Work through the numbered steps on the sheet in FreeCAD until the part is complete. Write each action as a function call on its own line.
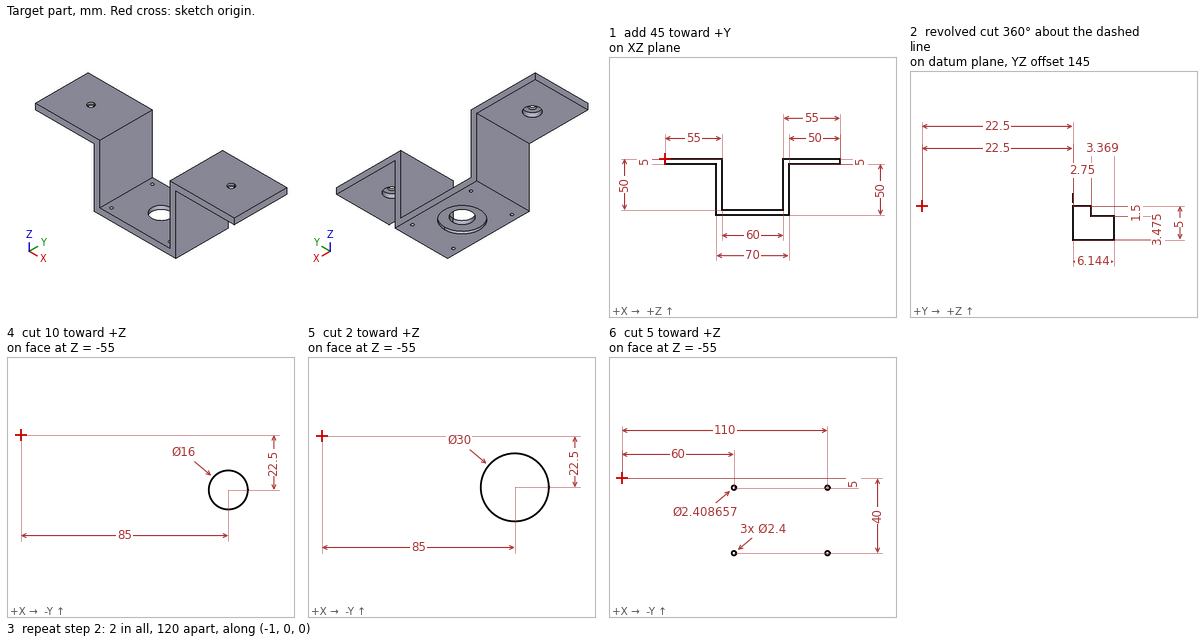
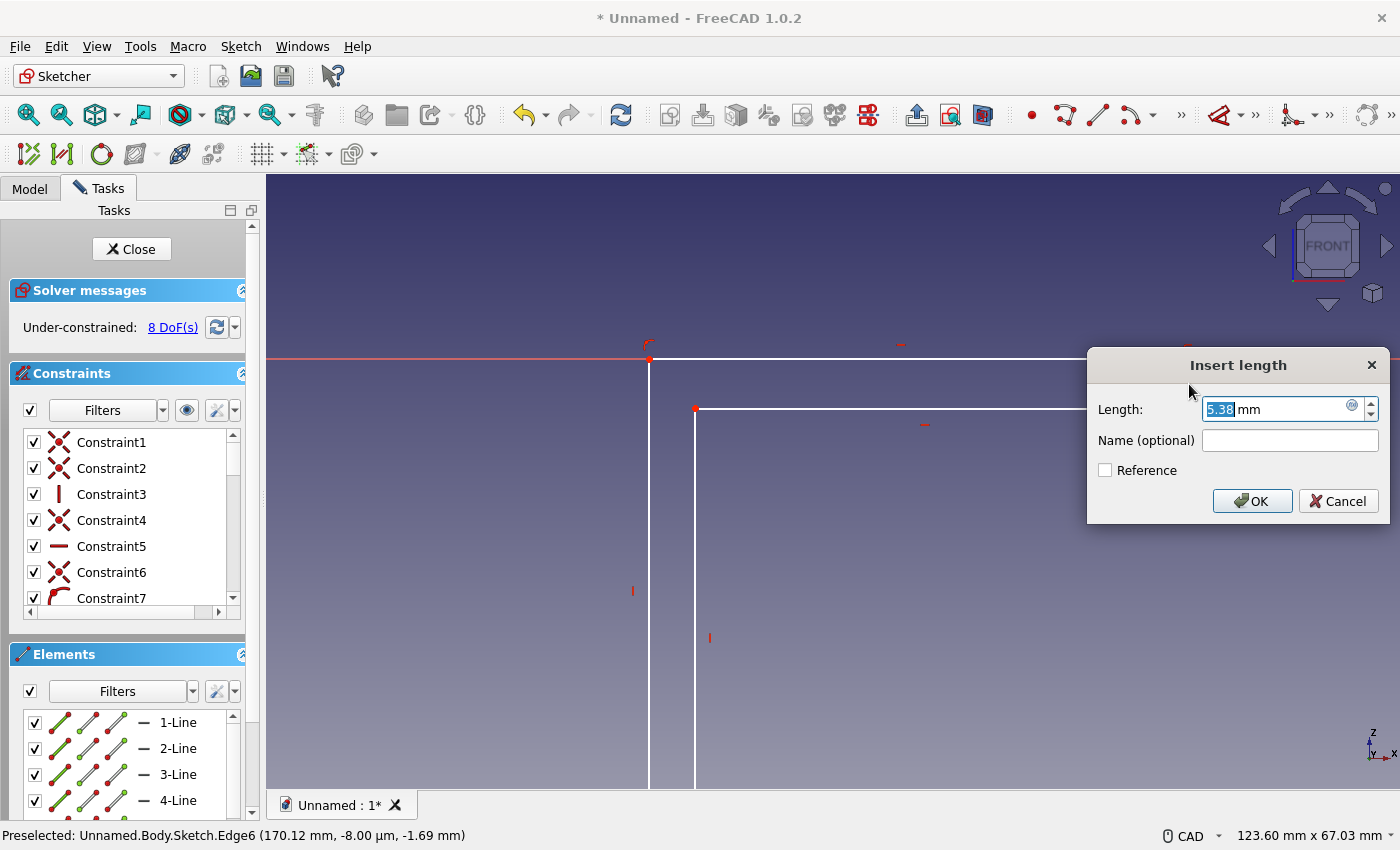
text(5)
key(Return)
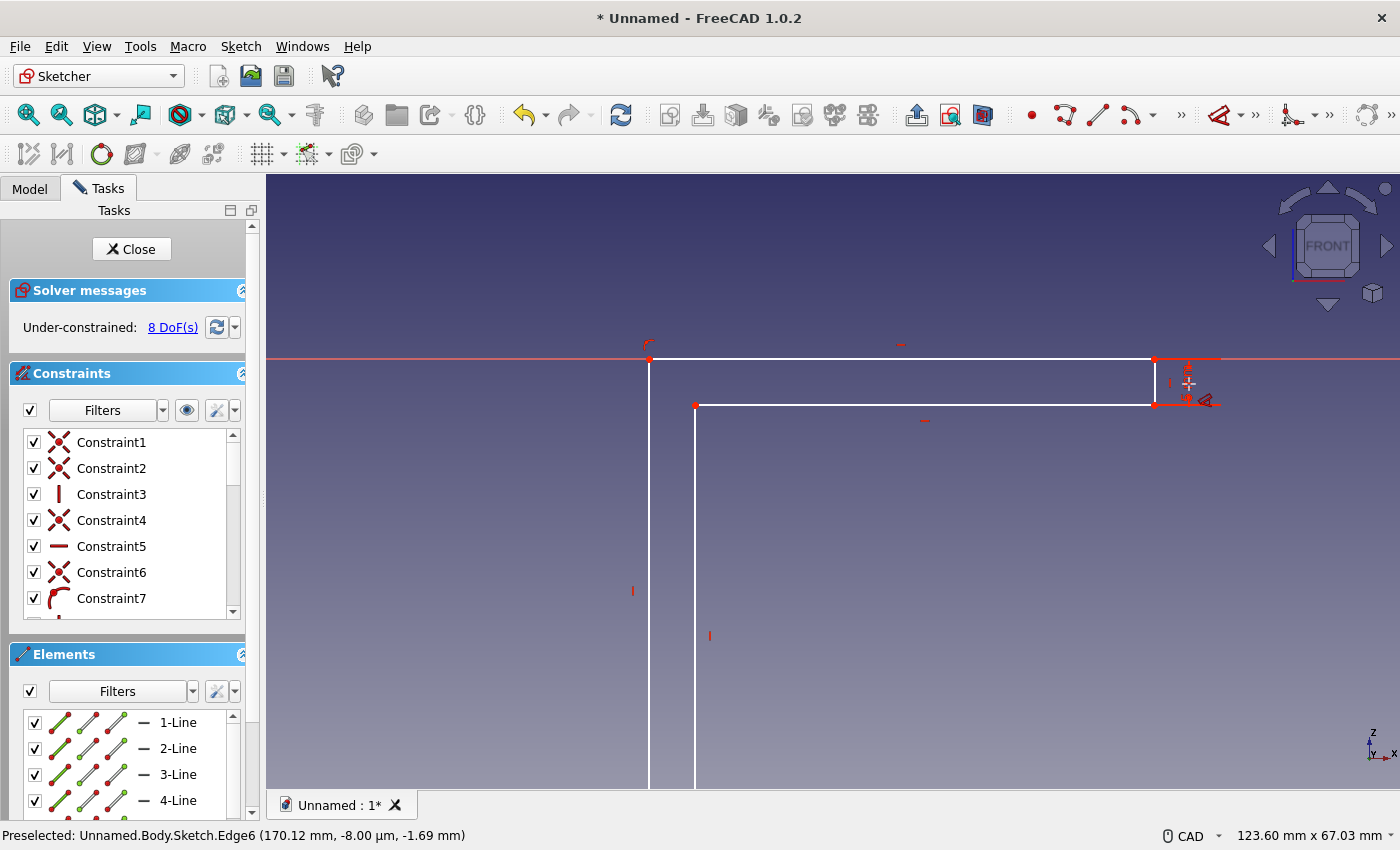
scroll(1083, 375, down, 4)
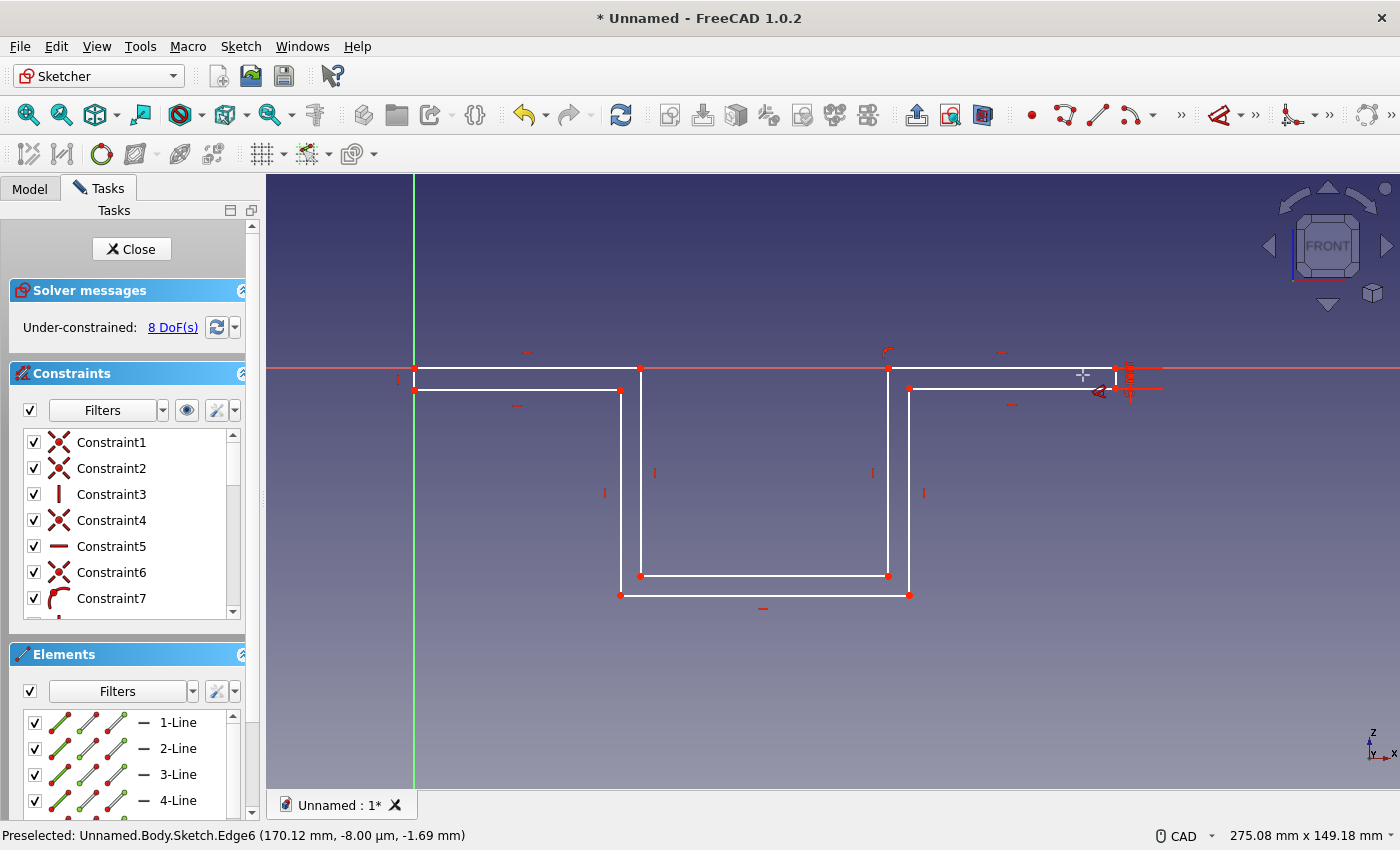
scroll(414, 384, up, 4)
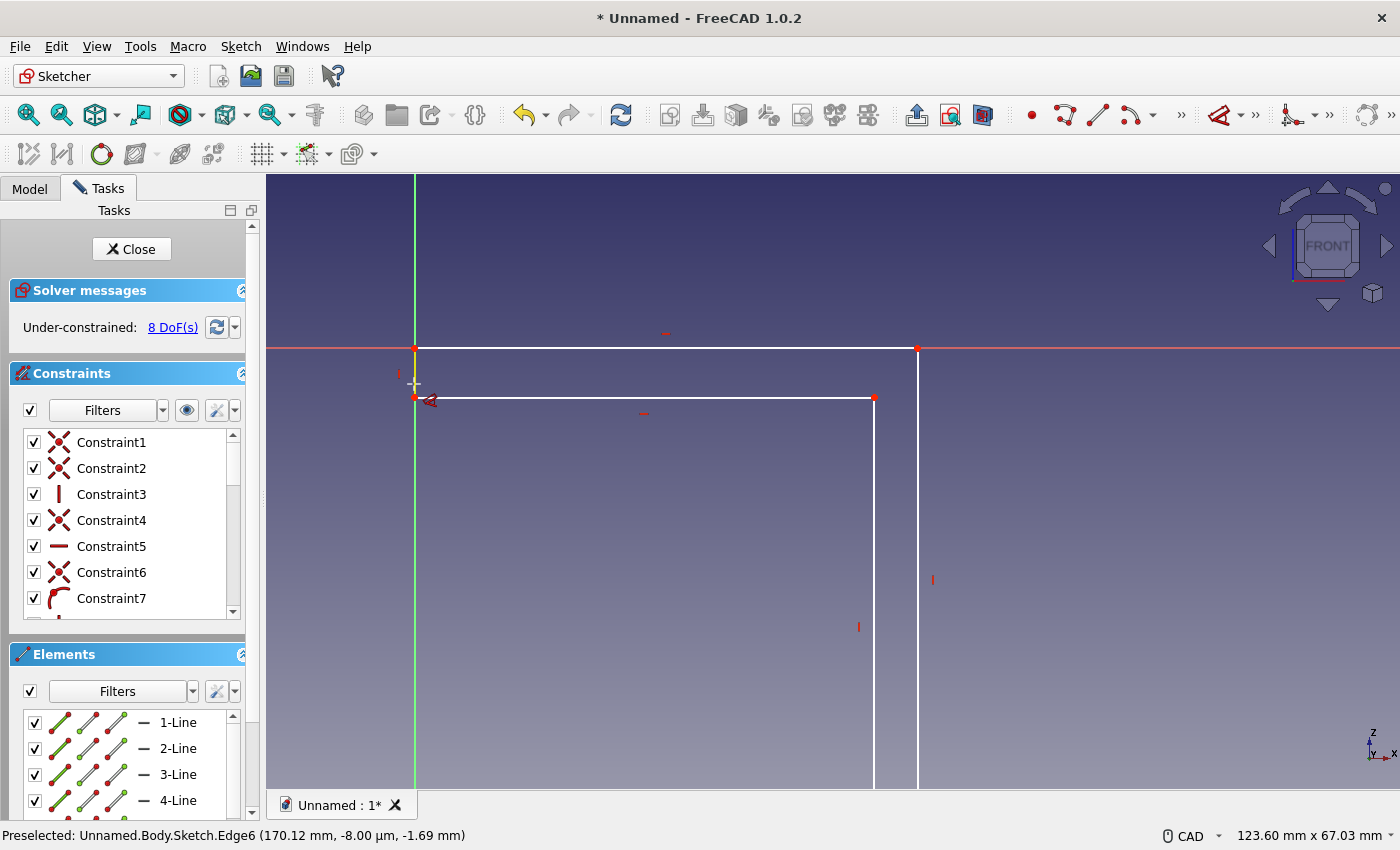
click(415, 383)
click(381, 373)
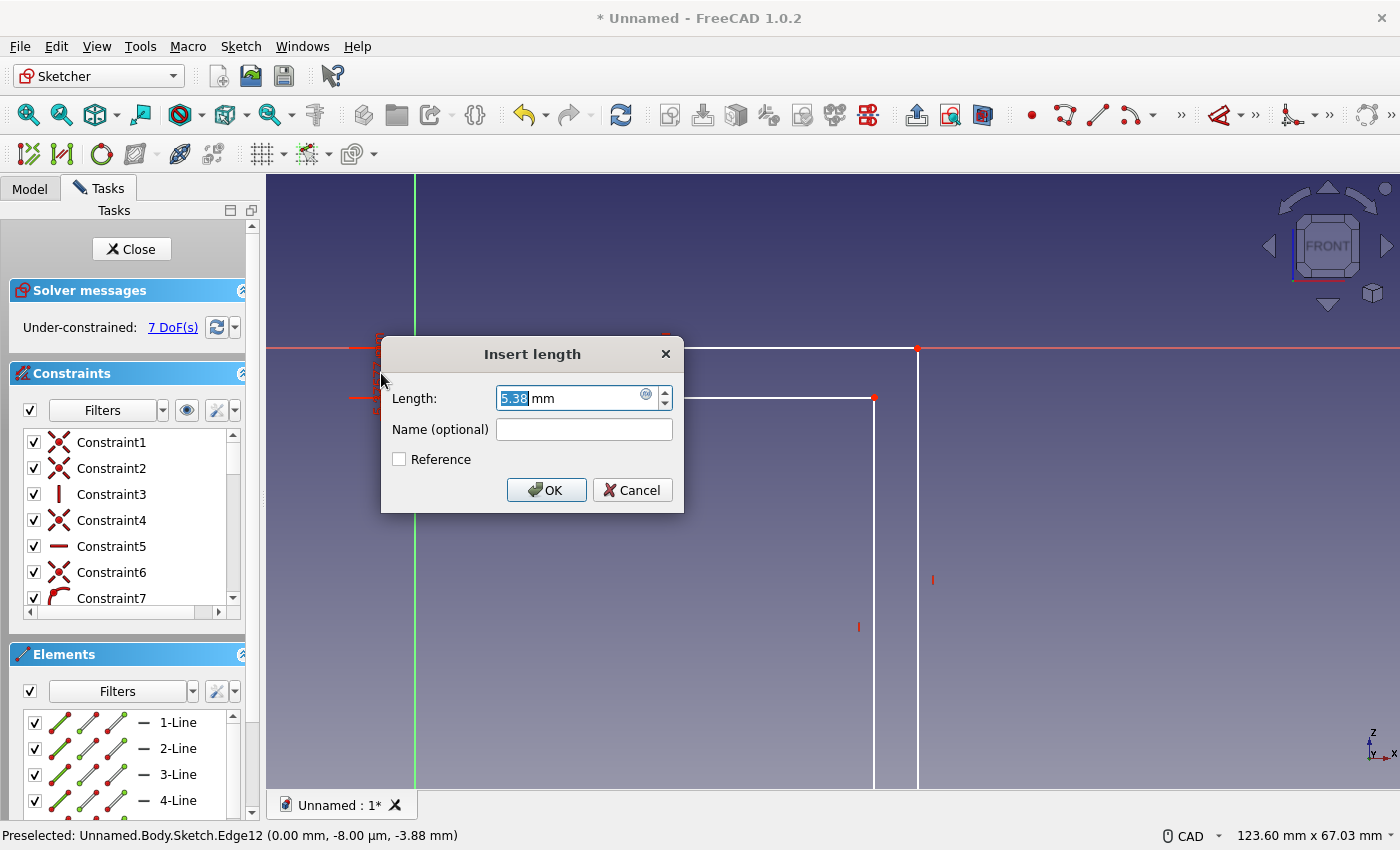
text(5)
key(Return)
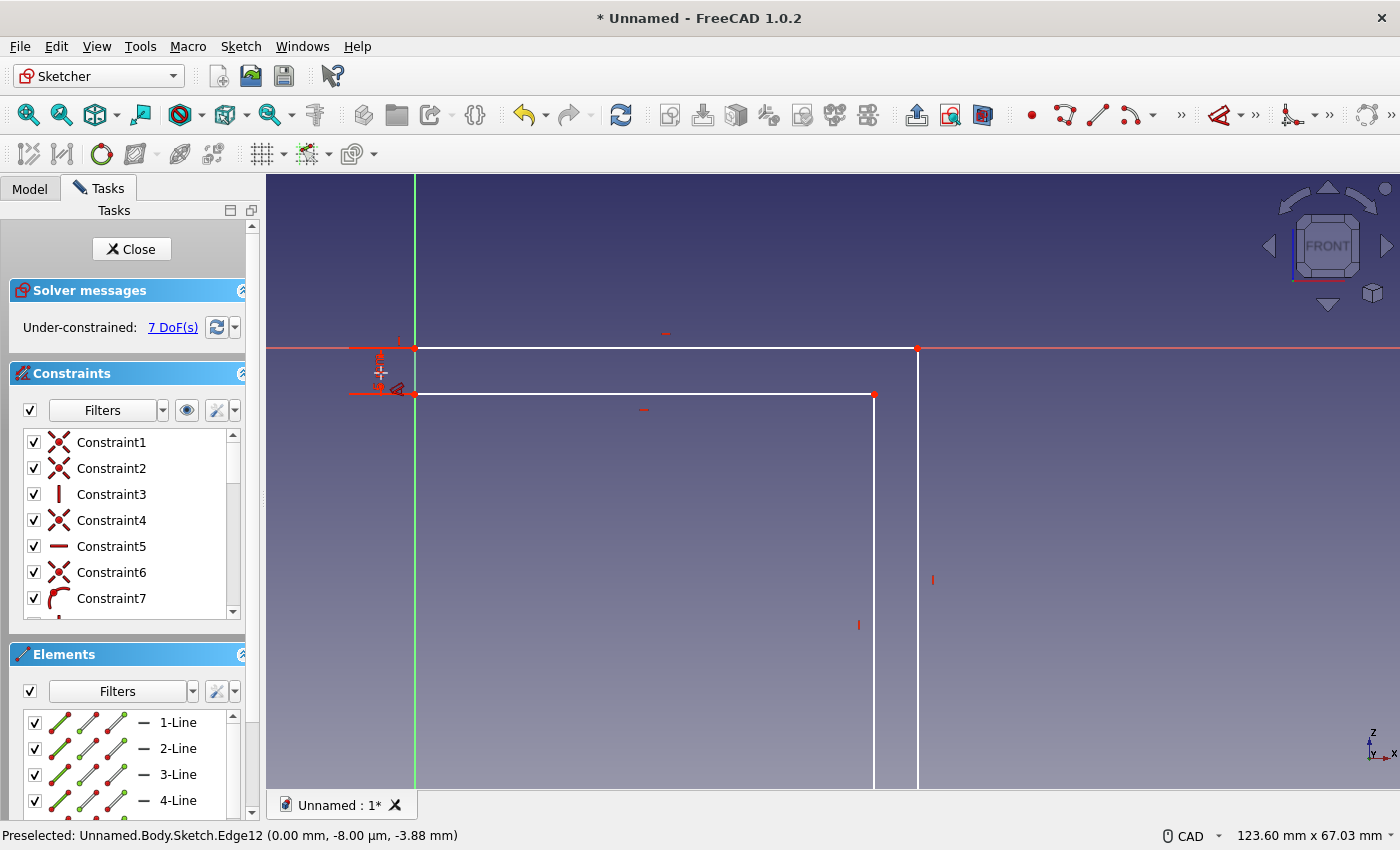
click(566, 348)
click(666, 314)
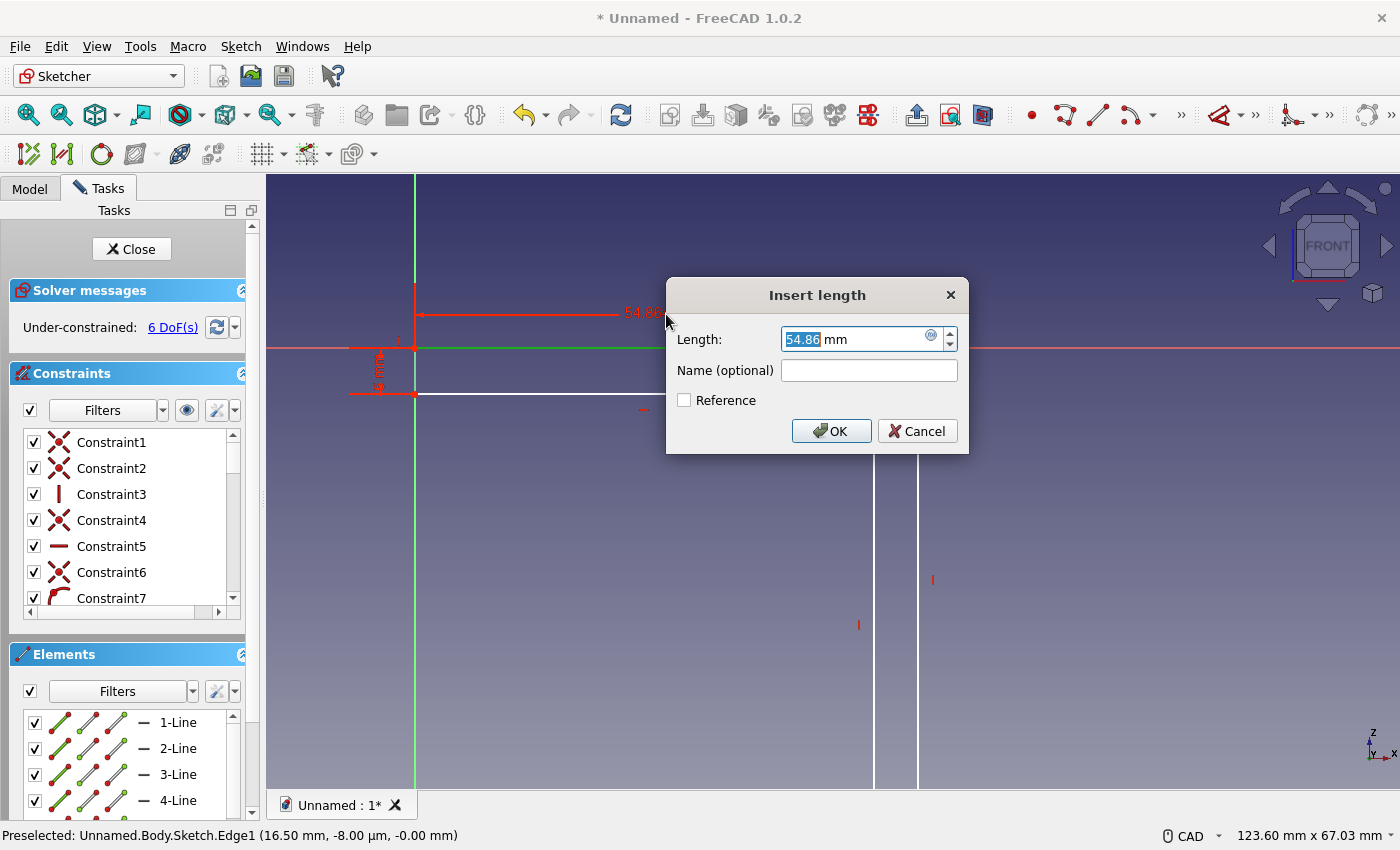
text(55)
key(Return)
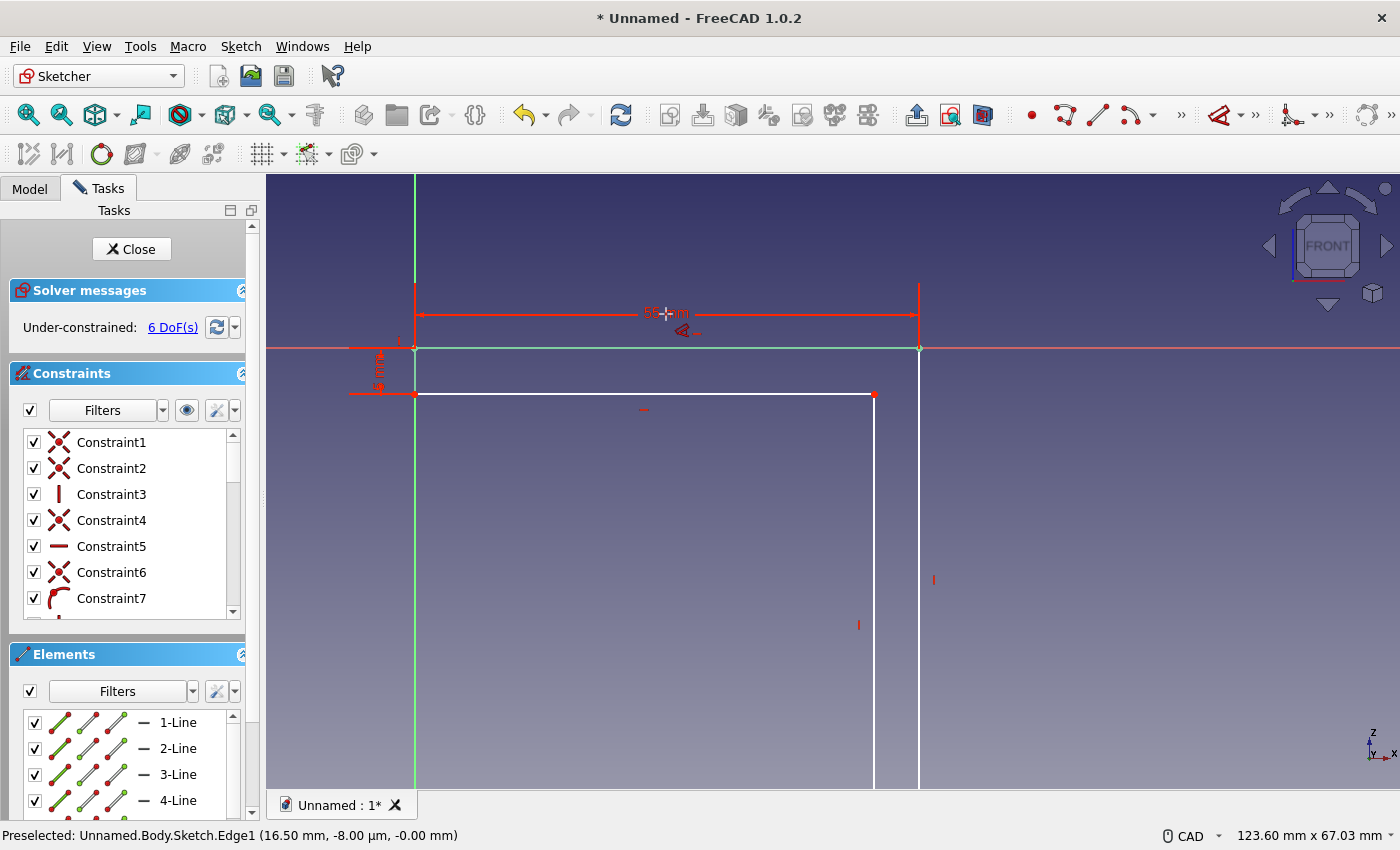
click(919, 487)
click(953, 555)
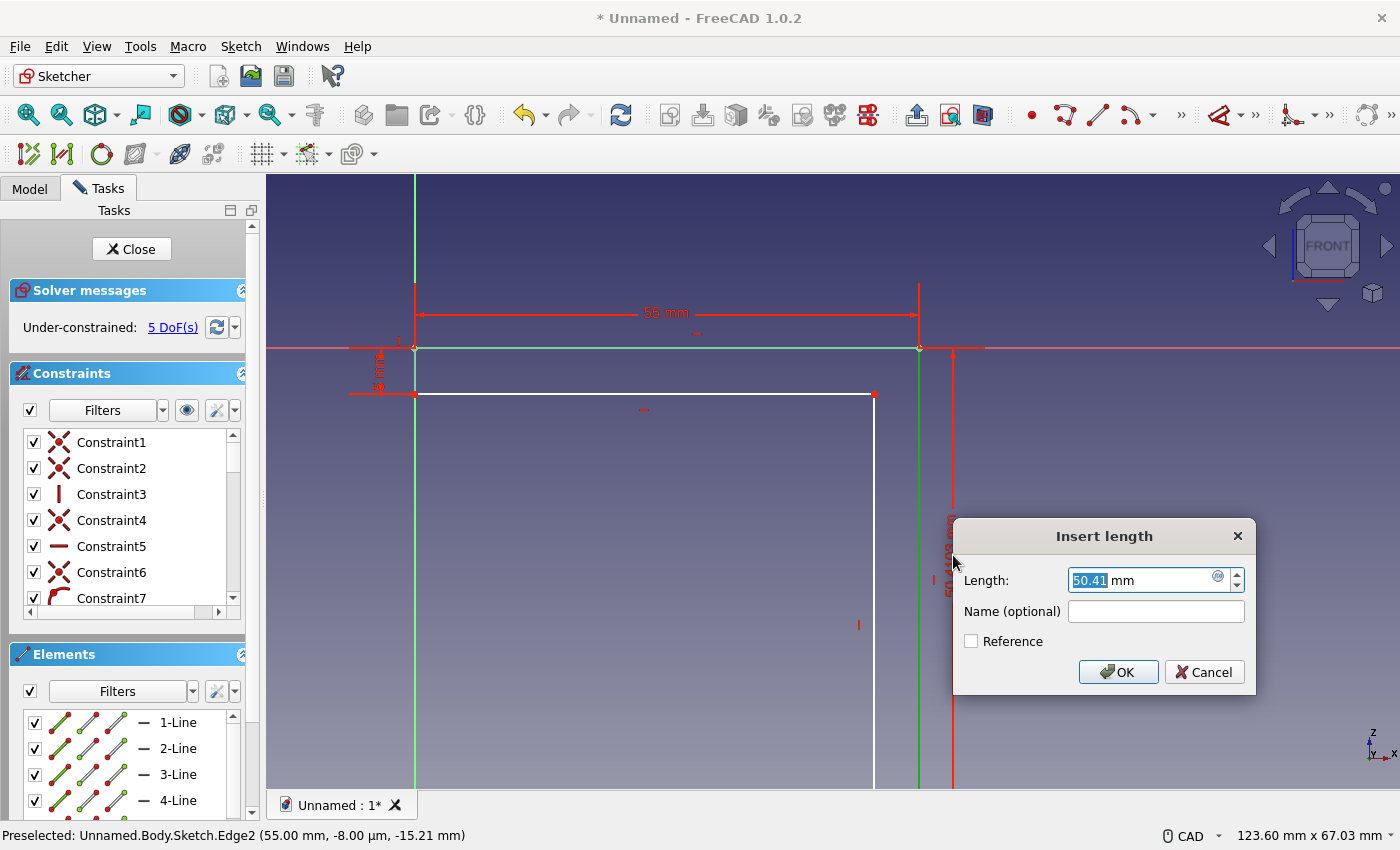
text(50)
key(Return)